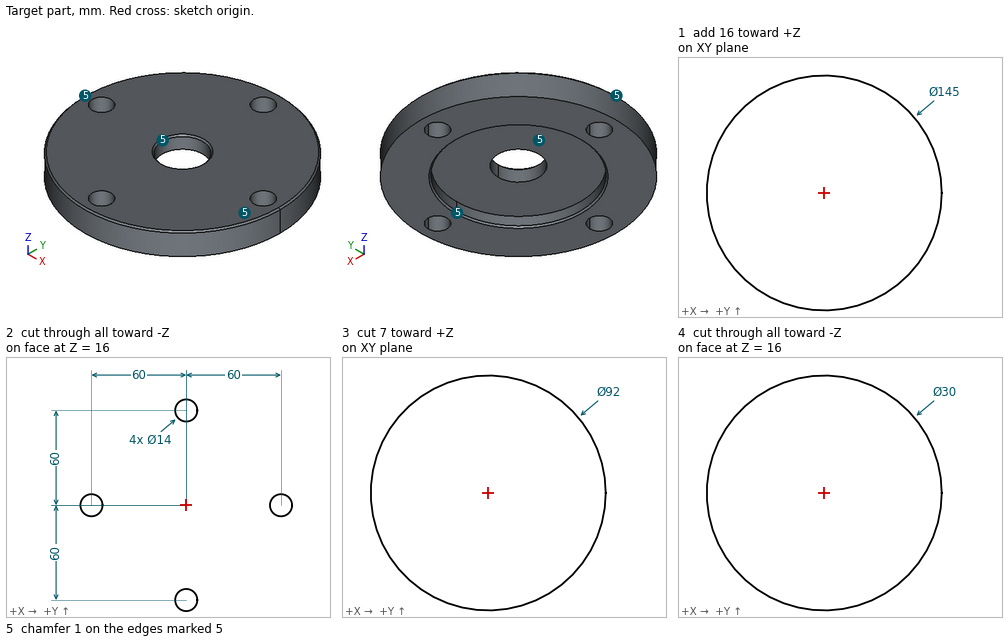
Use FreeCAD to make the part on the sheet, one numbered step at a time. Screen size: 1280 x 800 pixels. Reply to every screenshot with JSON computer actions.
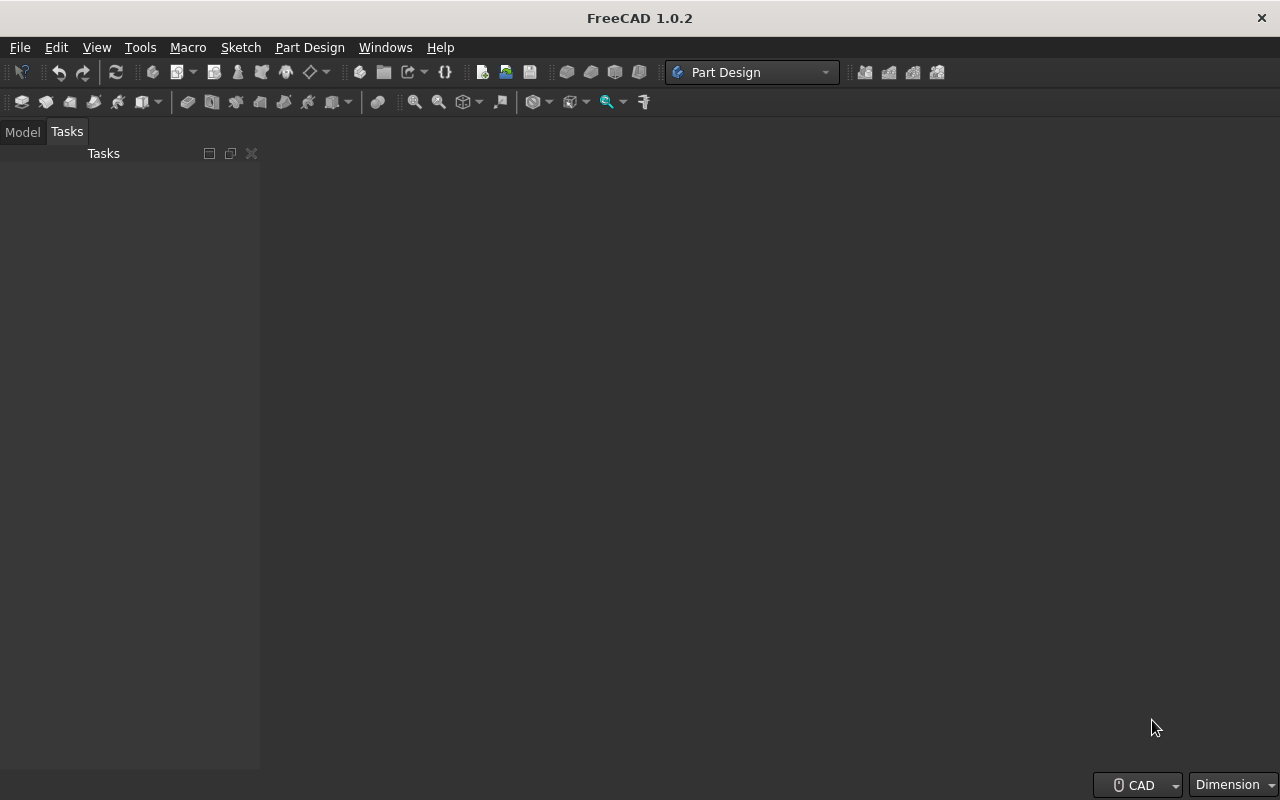
{"action": "key", "text": "ctrl+n"}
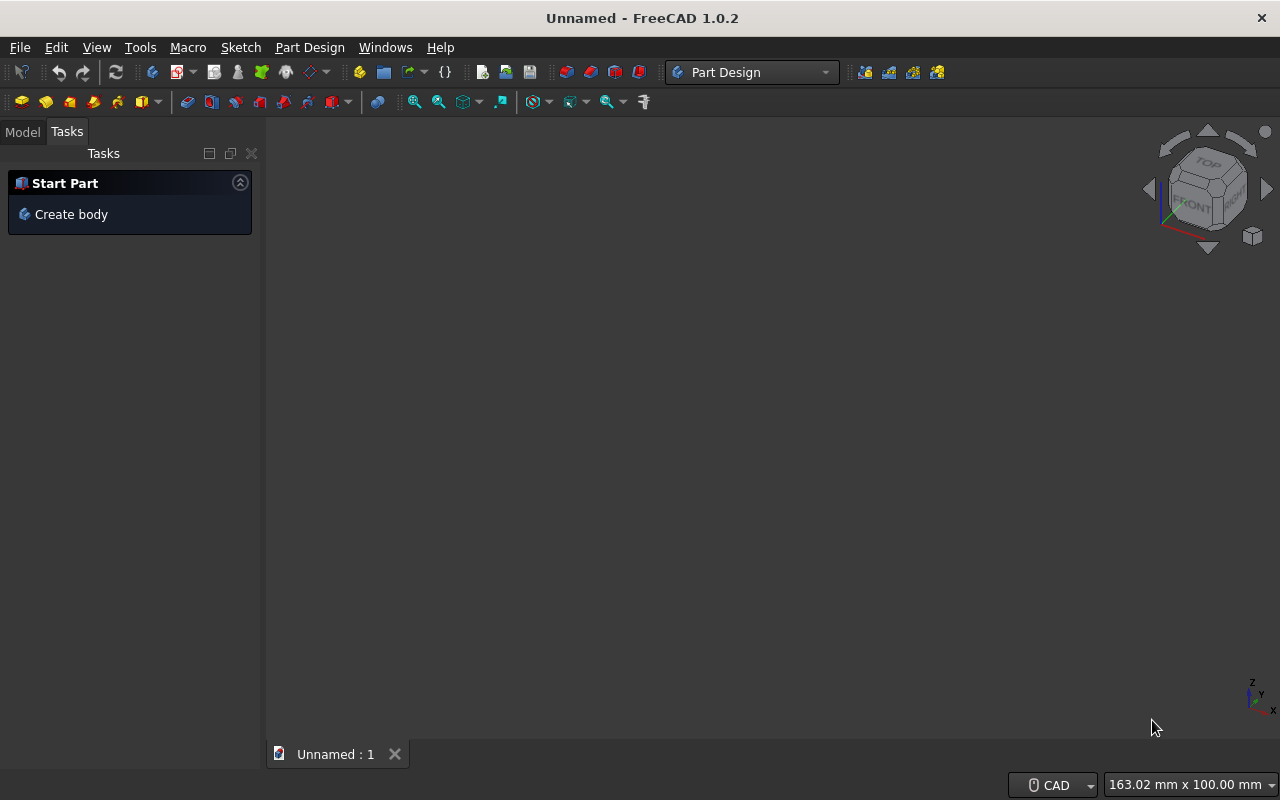
{"action": "left_click", "coordinate": [178, 72]}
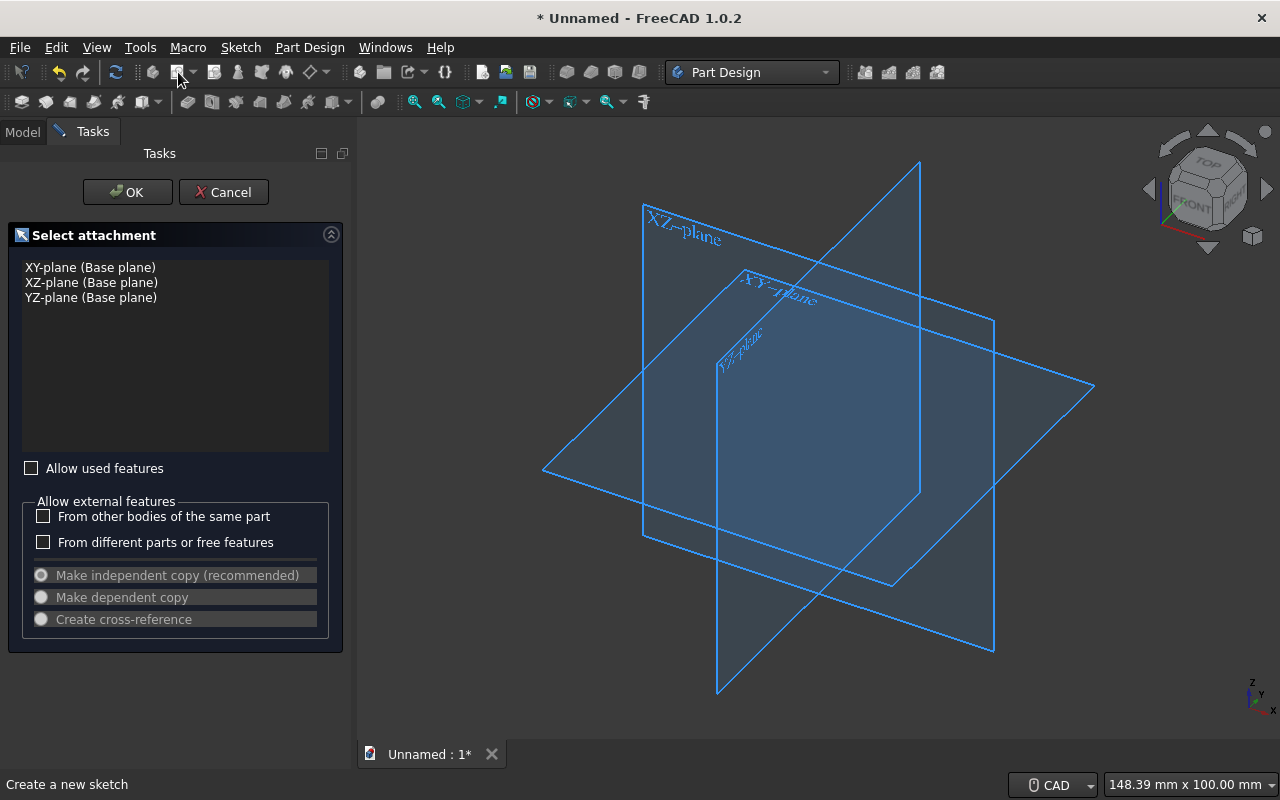
{"action": "left_click", "coordinate": [82, 268]}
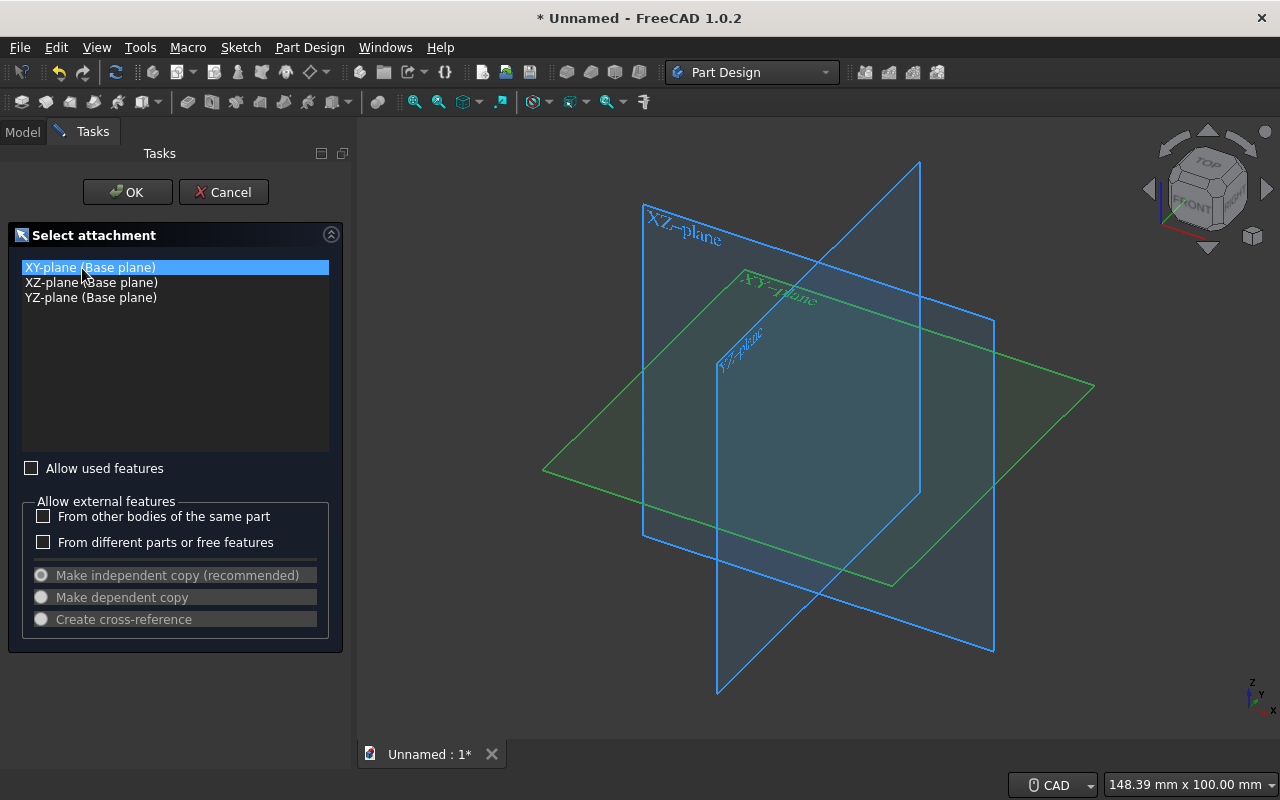
{"action": "left_click", "coordinate": [128, 192]}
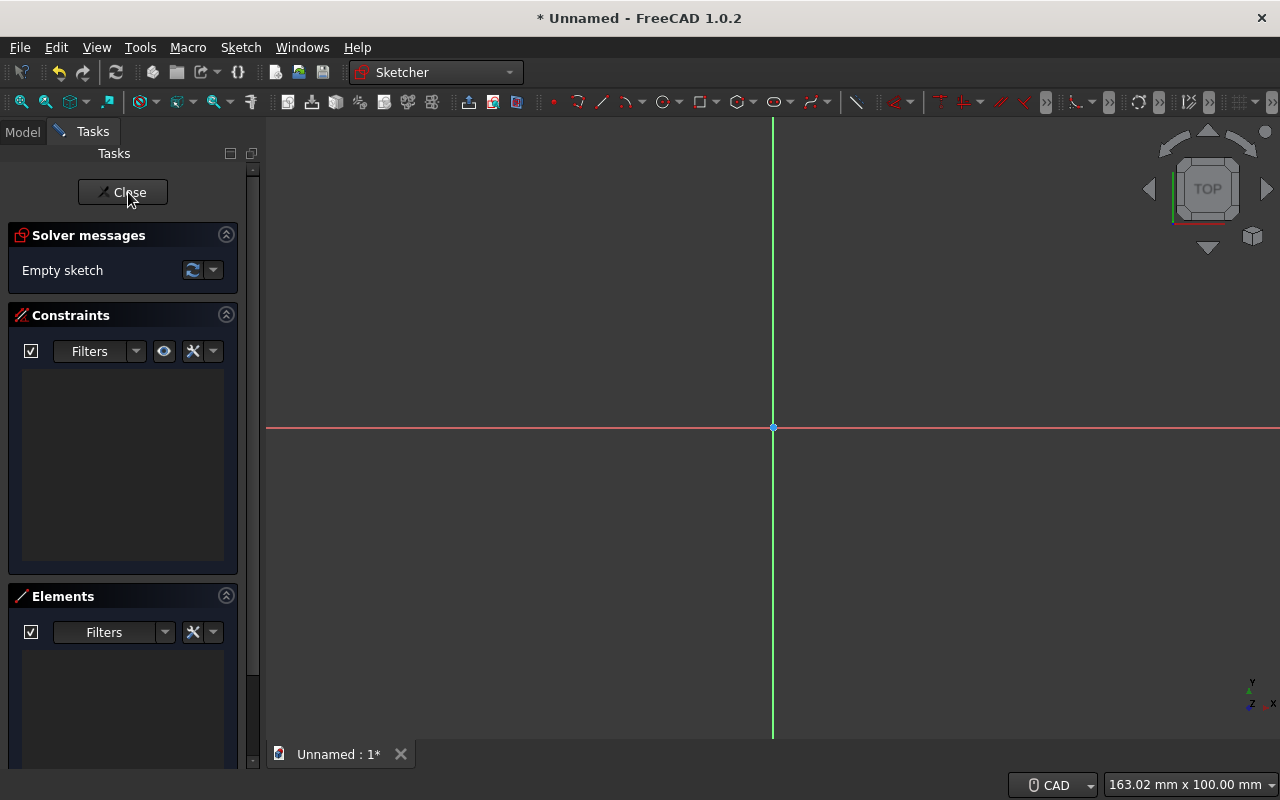
{"action": "scroll", "coordinate": [649, 428], "scroll_direction": "down", "scroll_amount": 4}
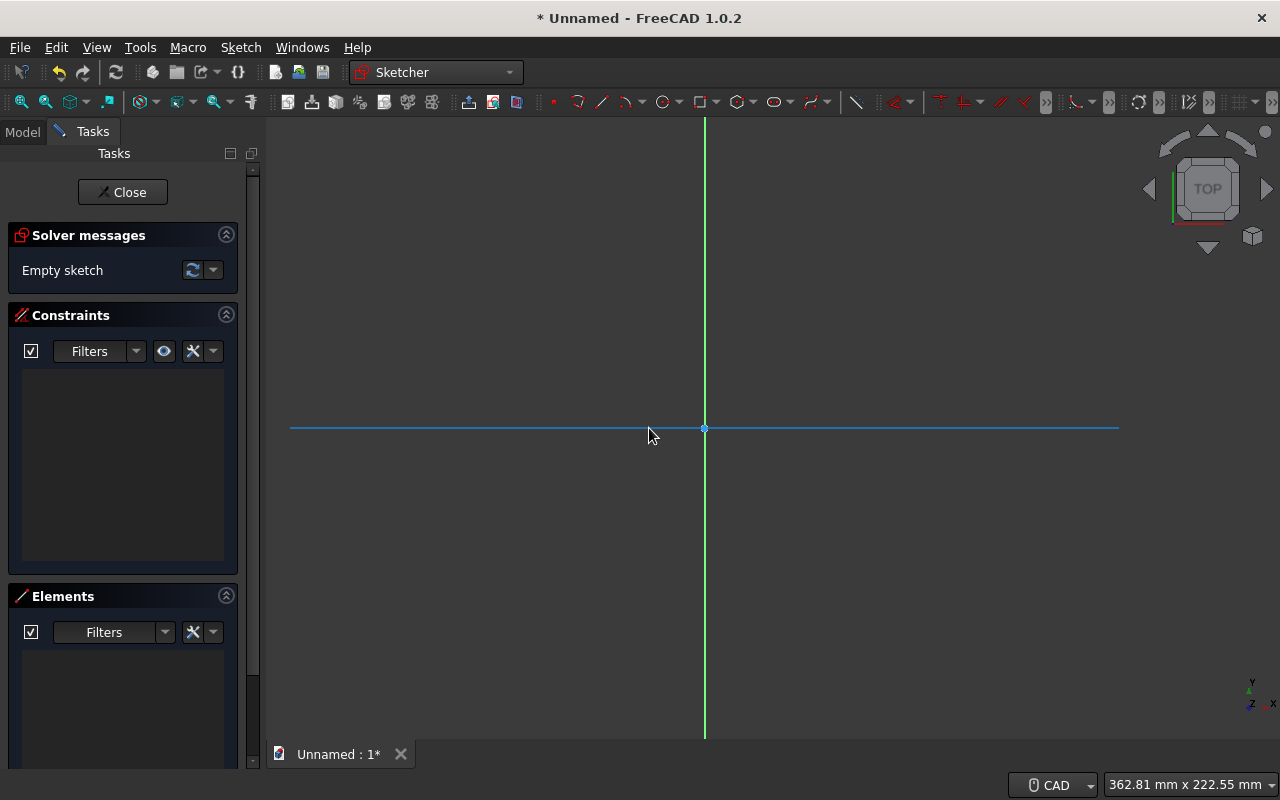
{"action": "key", "text": "g c"}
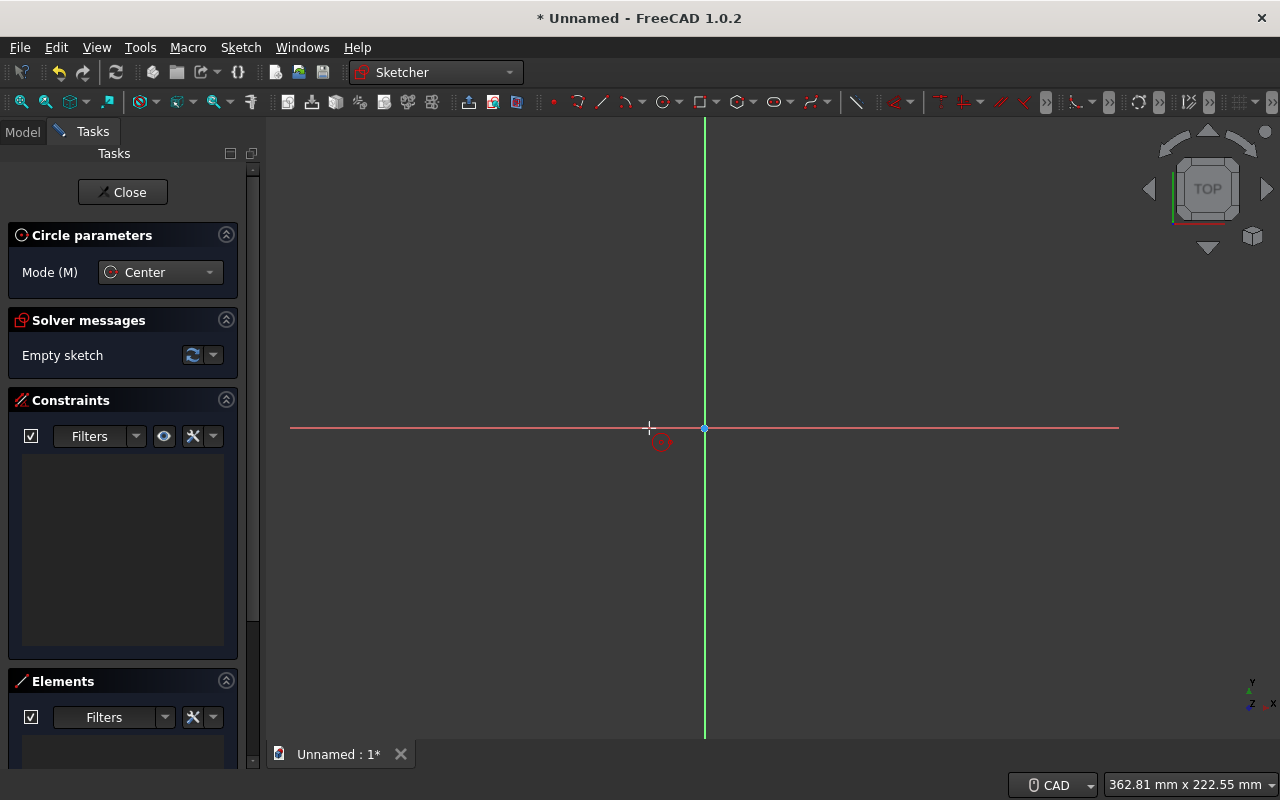
{"action": "left_click", "coordinate": [705, 428]}
{"action": "left_click", "coordinate": [848, 285]}
{"action": "key", "text": "Escape"}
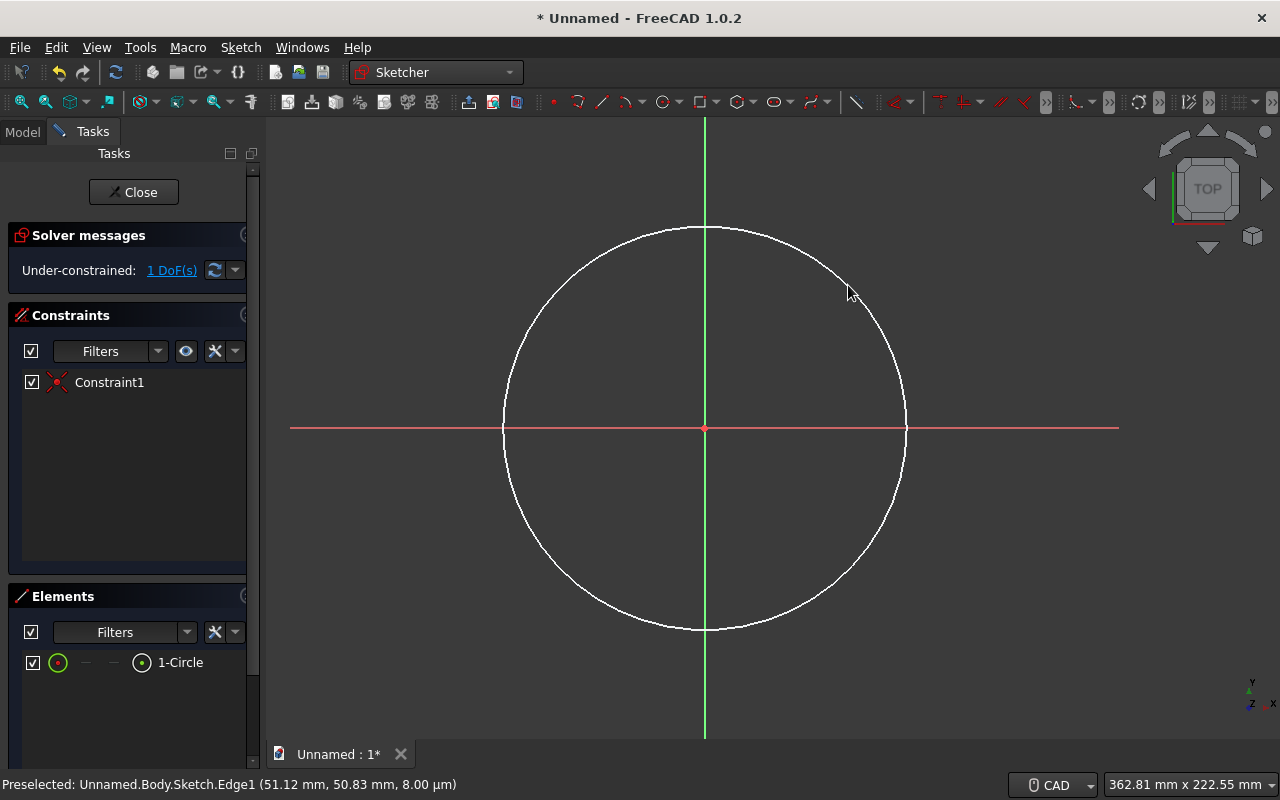
{"action": "key", "text": "d"}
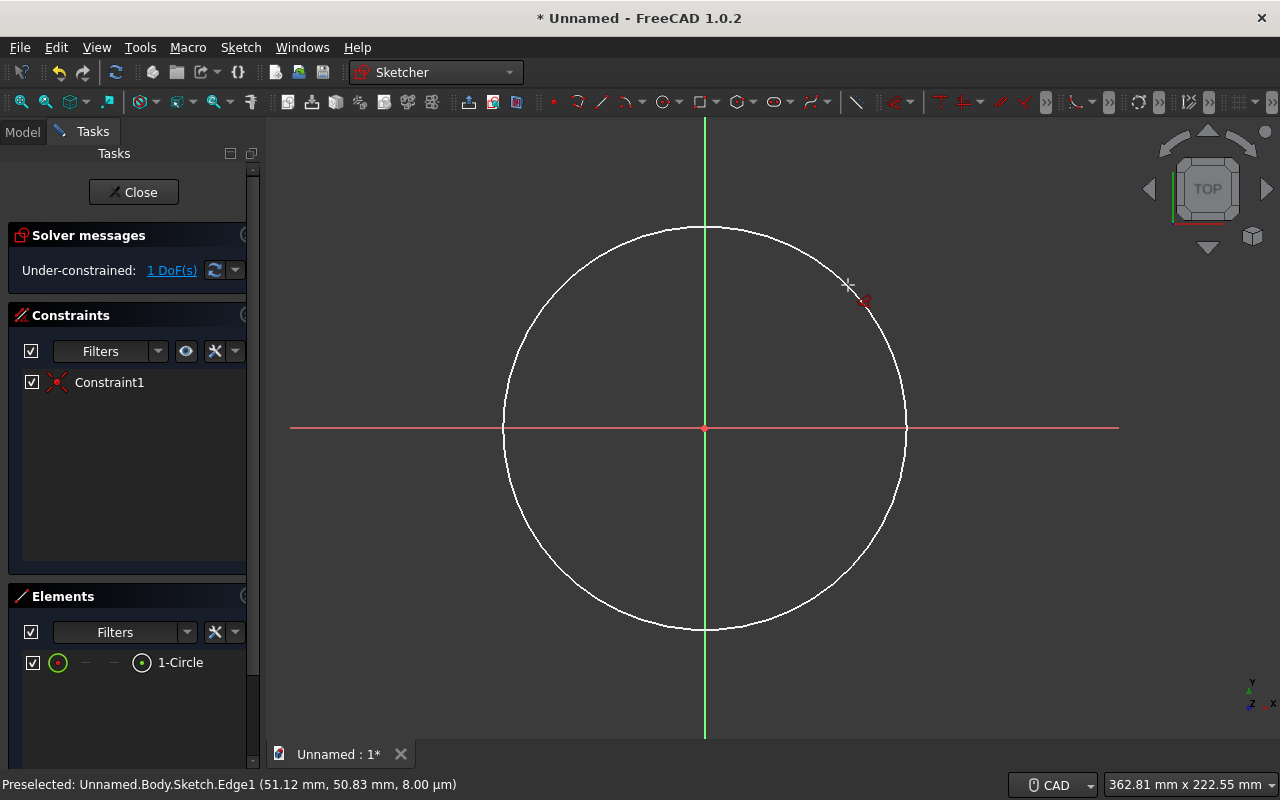
{"action": "left_click", "coordinate": [847, 285]}
{"action": "left_click", "coordinate": [870, 262]}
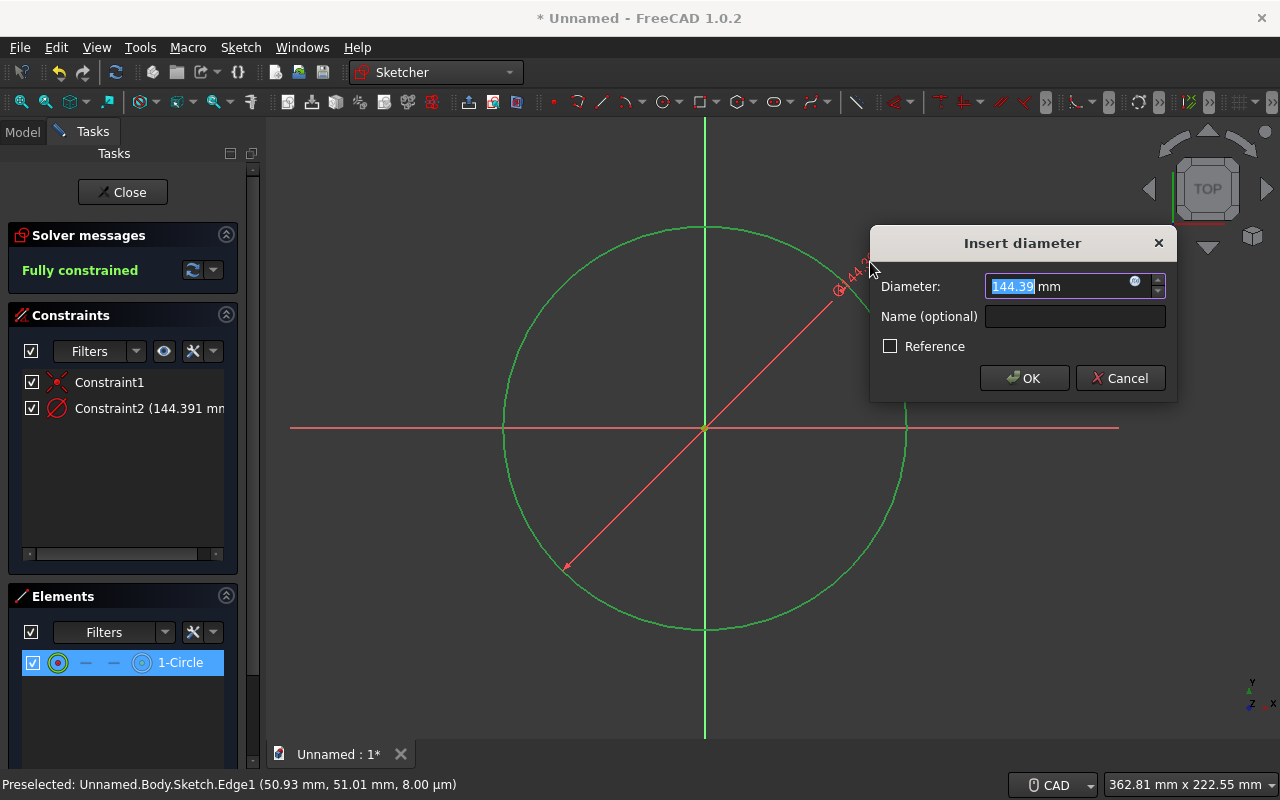
{"action": "type", "text": "145"}
{"action": "key", "text": "Return"}
{"action": "key", "text": "Escape"}